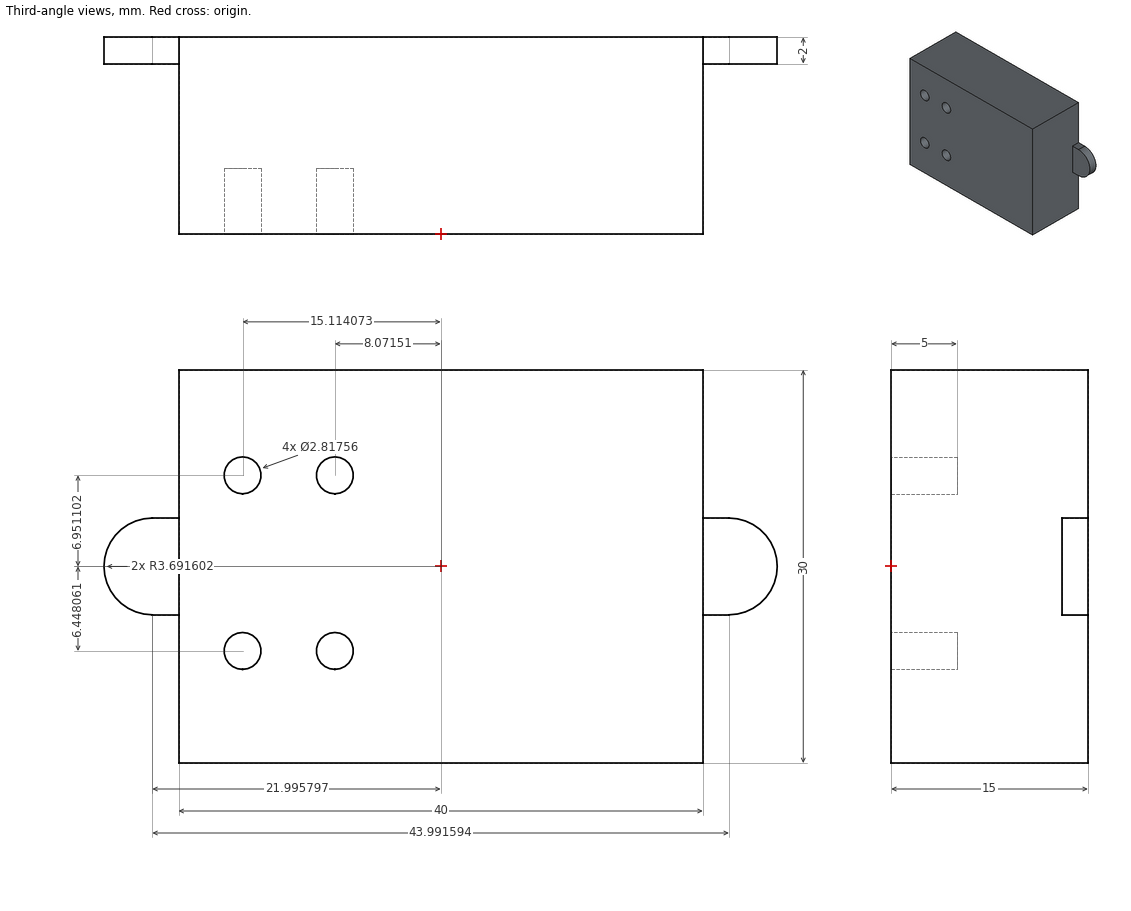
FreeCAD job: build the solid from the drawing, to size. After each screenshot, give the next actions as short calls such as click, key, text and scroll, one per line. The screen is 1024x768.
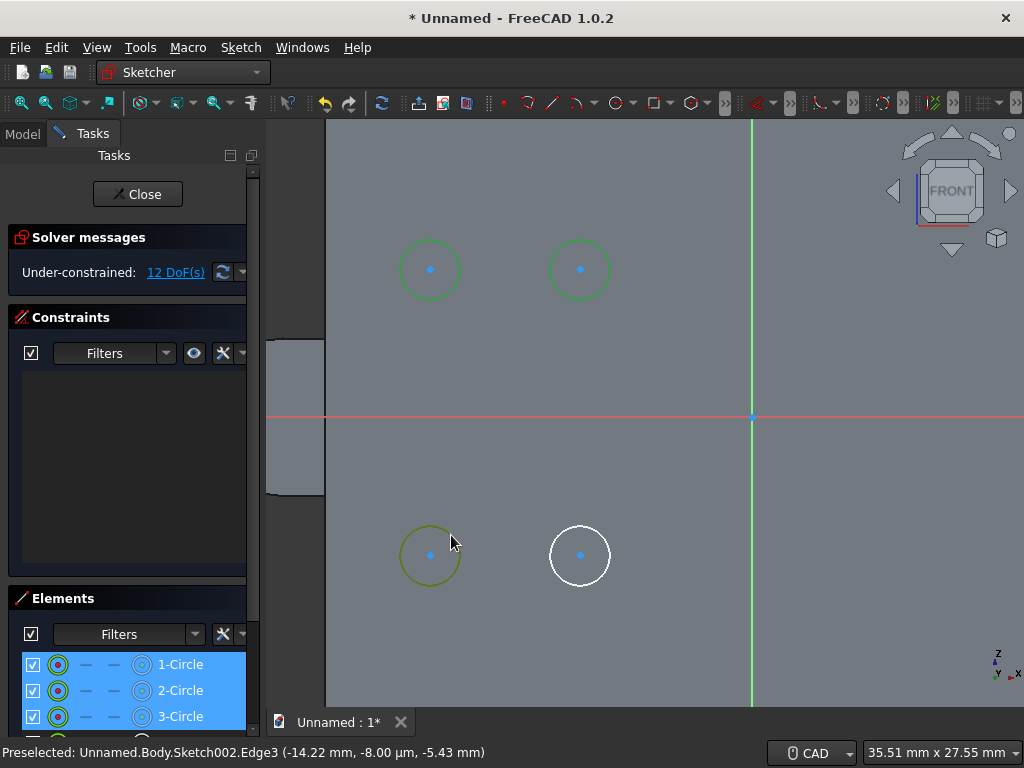
click(601, 535)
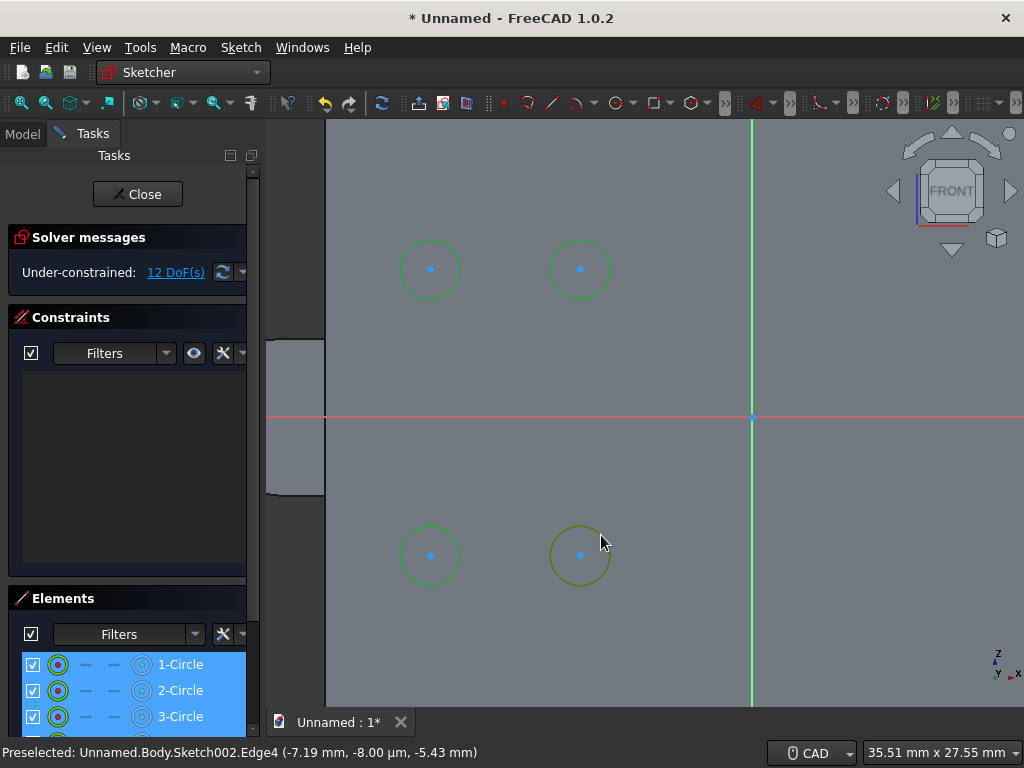
key(e)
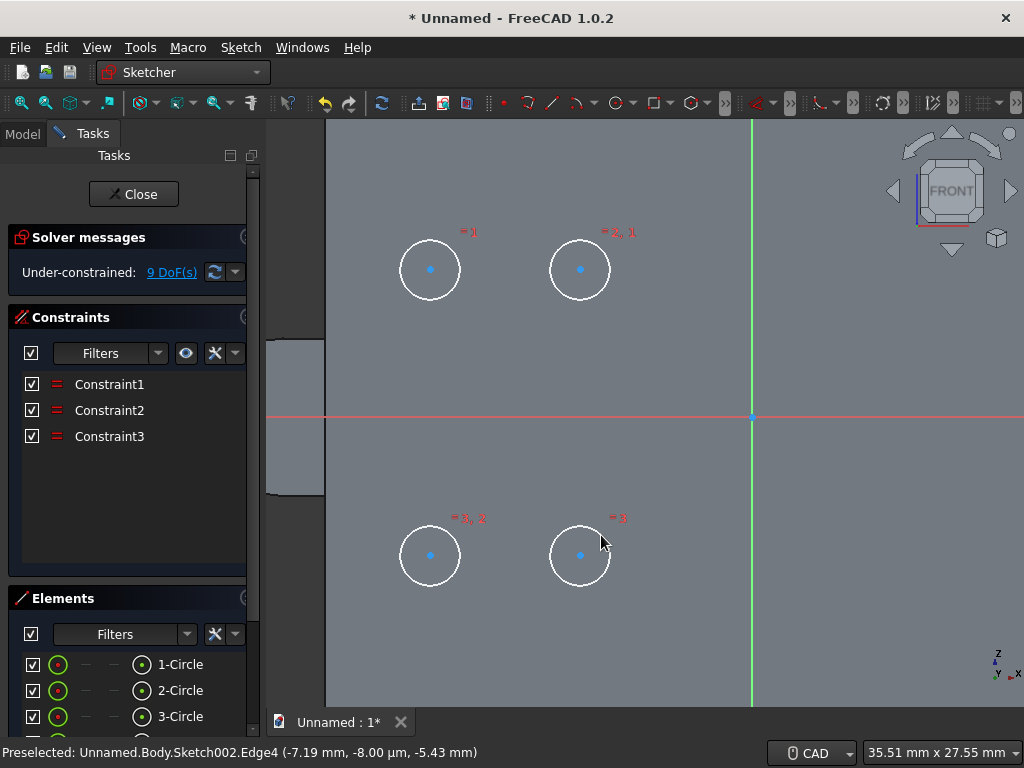
key(d)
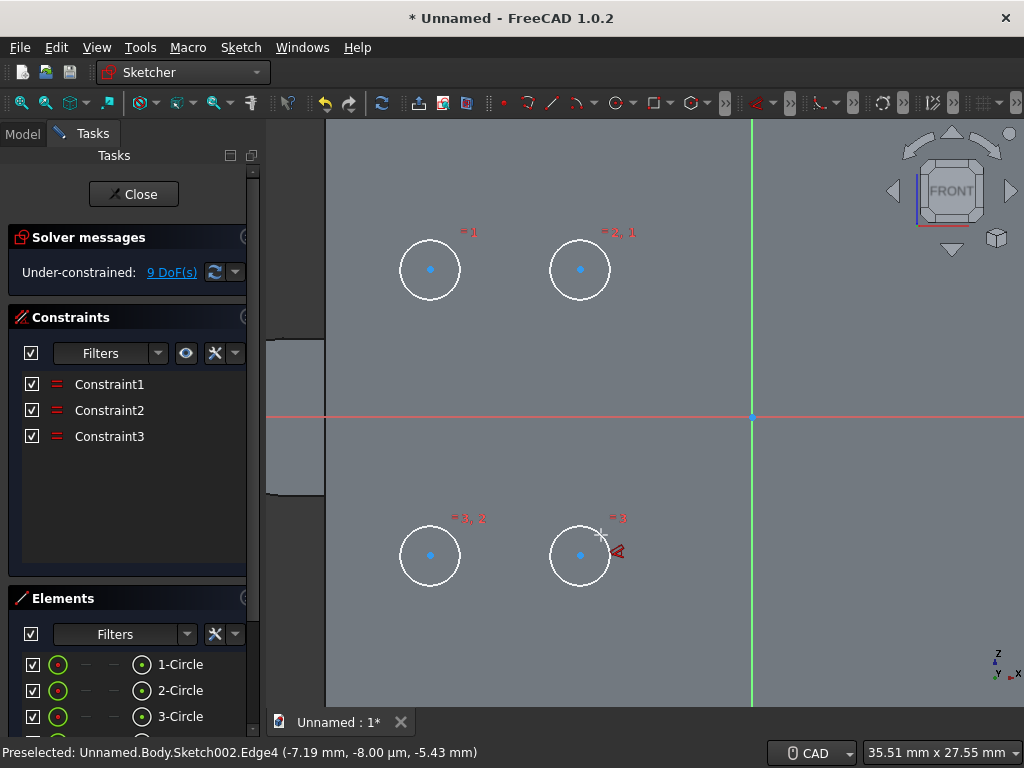
click(451, 249)
click(474, 226)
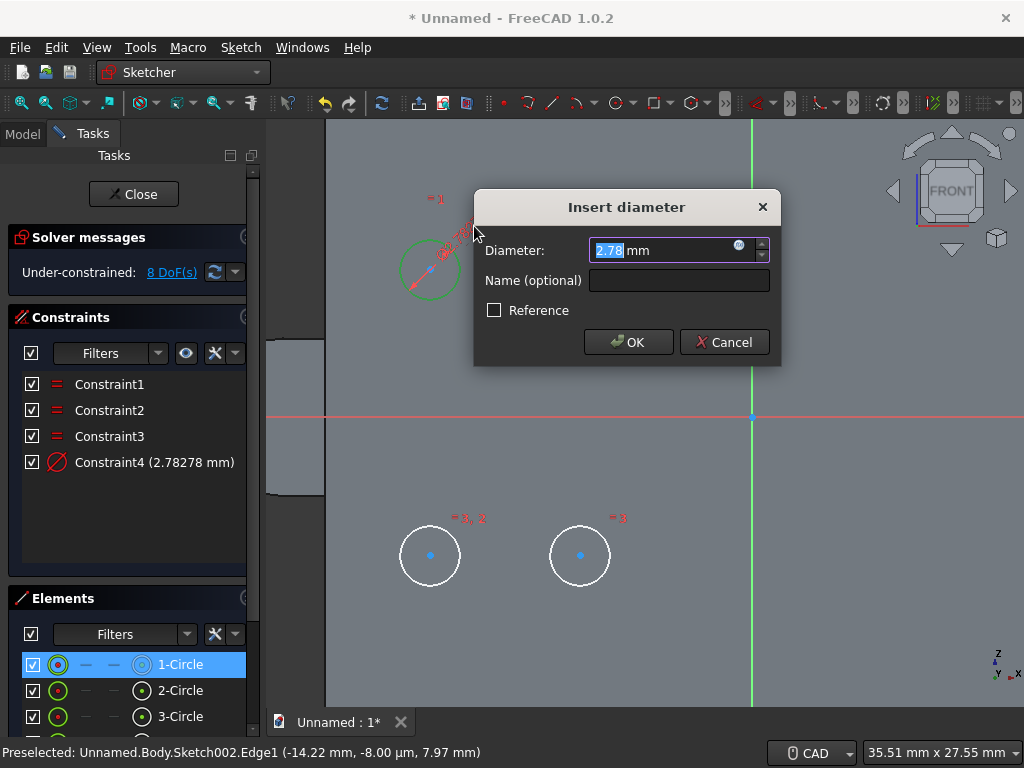
text(2.81756)
key(Return)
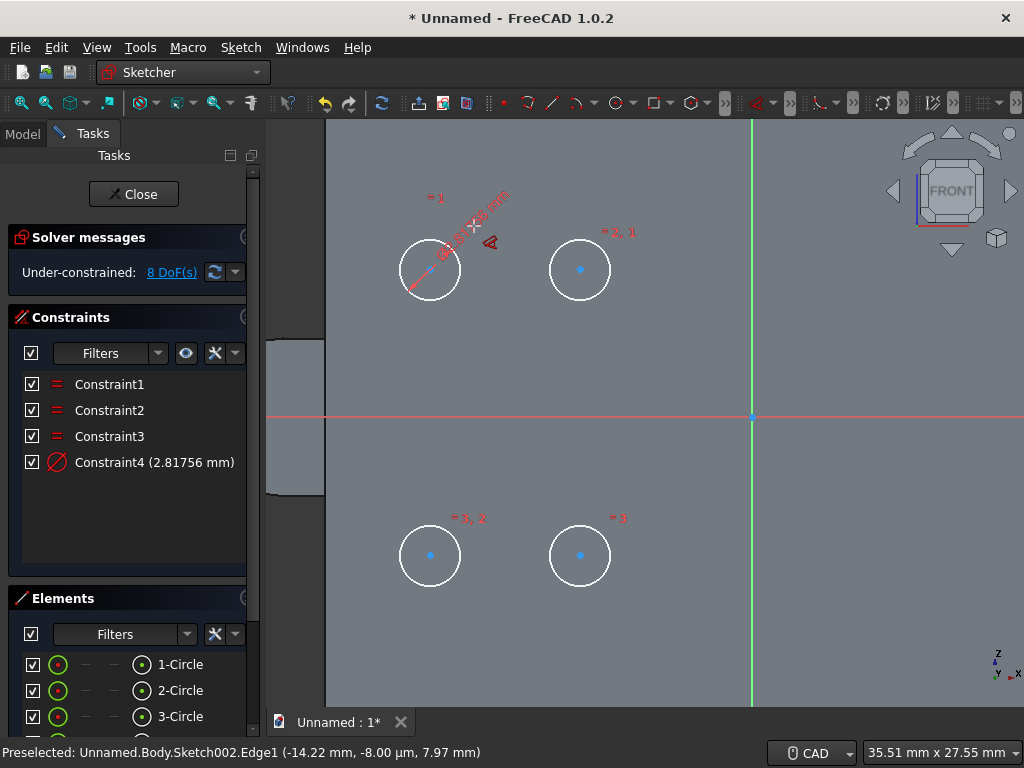
click(580, 270)
click(666, 236)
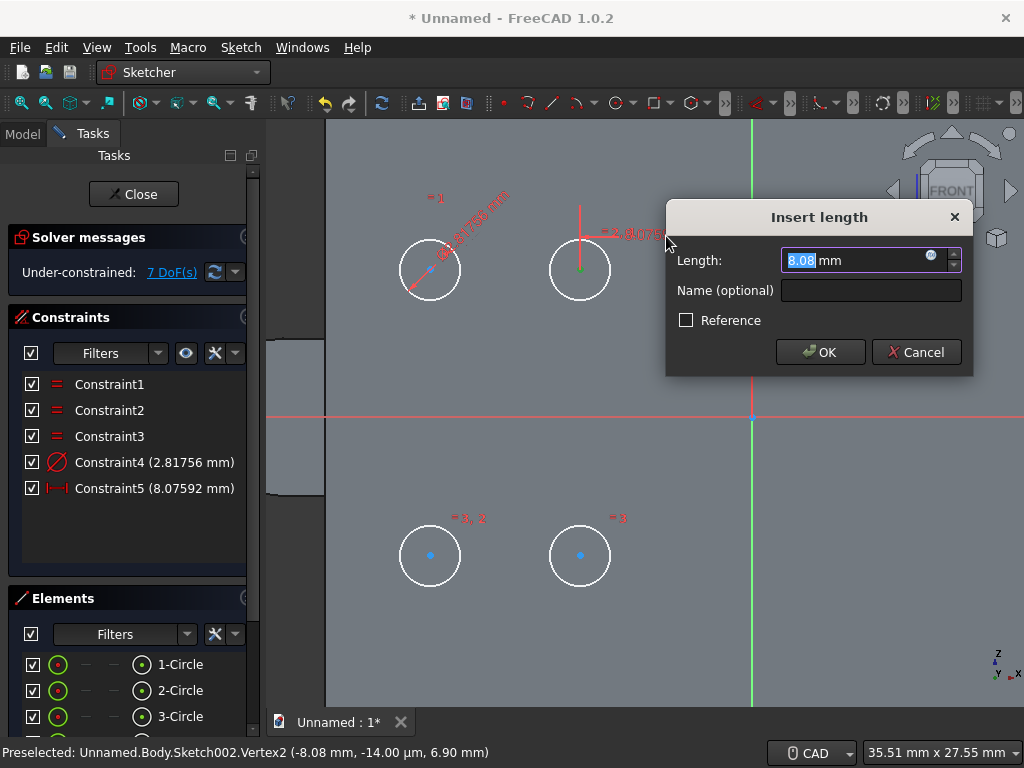
text(8.07151)
key(Return)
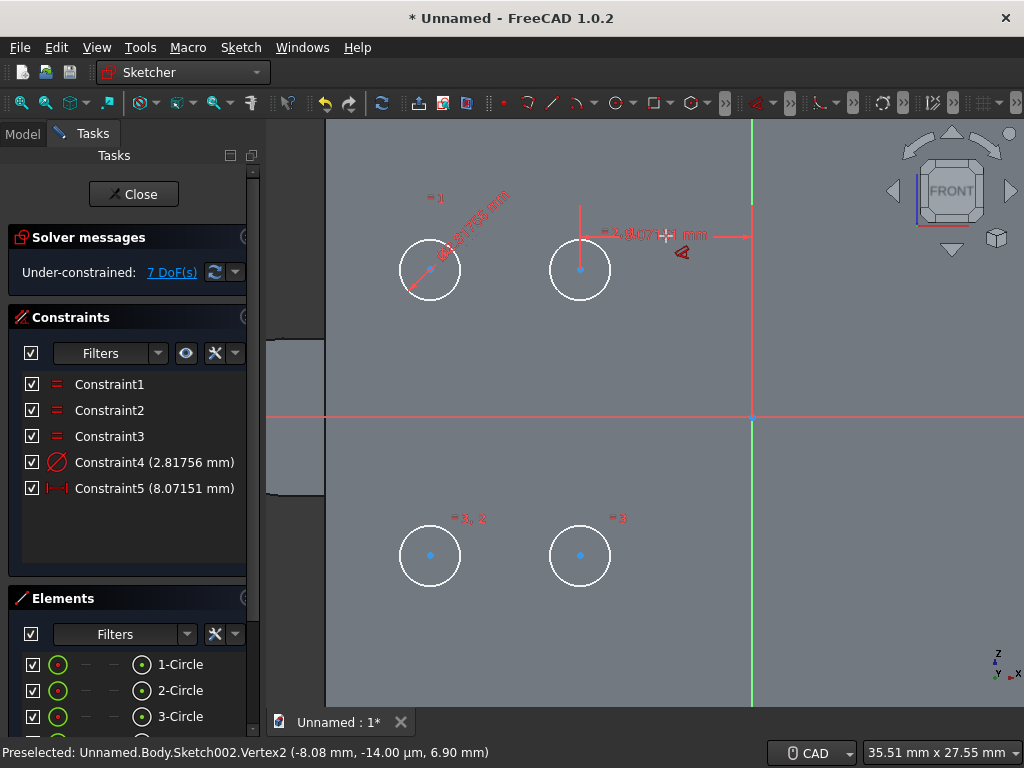
click(580, 556)
click(666, 590)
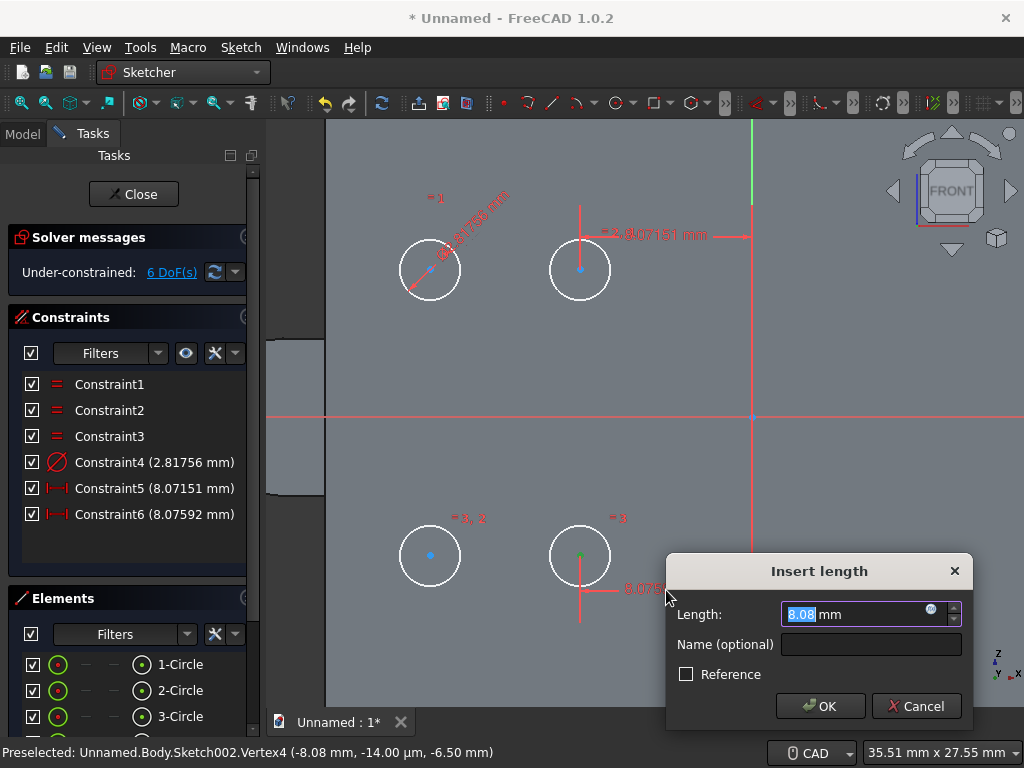
text(8.07151)
key(Return)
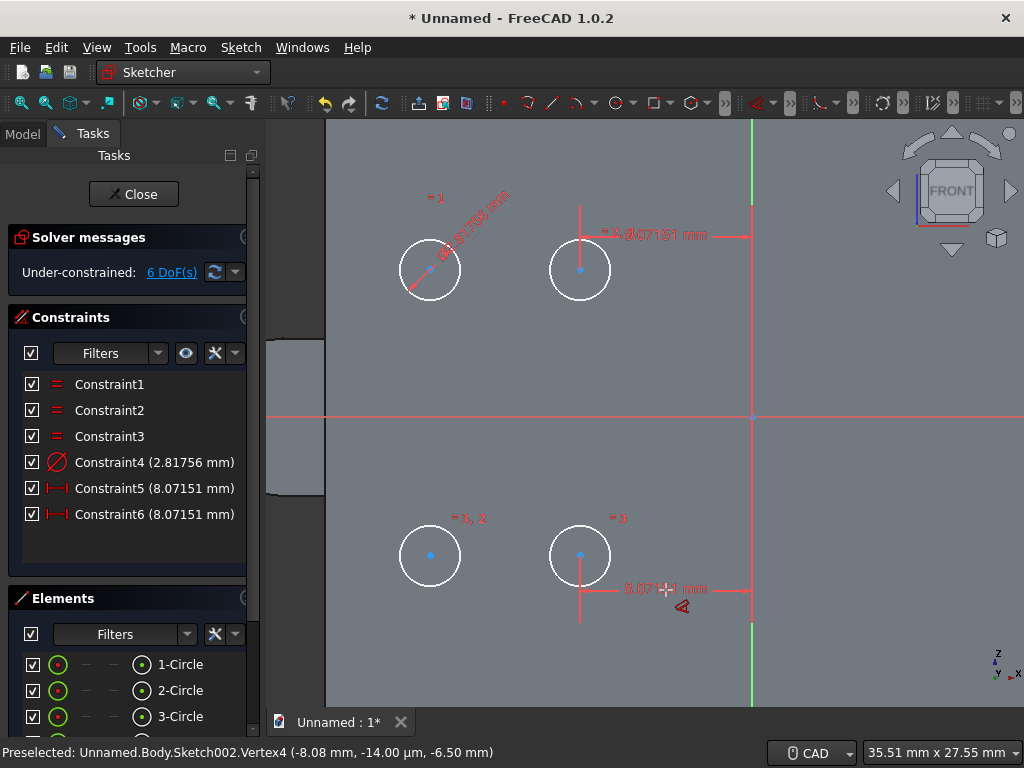
click(430, 270)
click(786, 344)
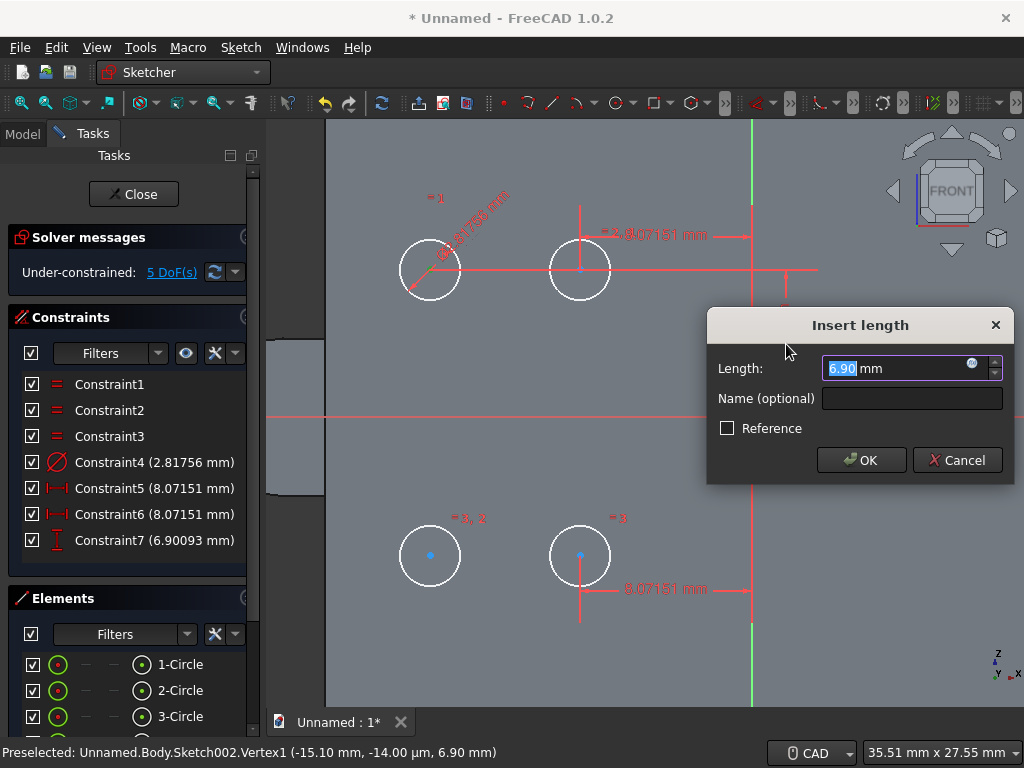
text(6.951102)
key(Return)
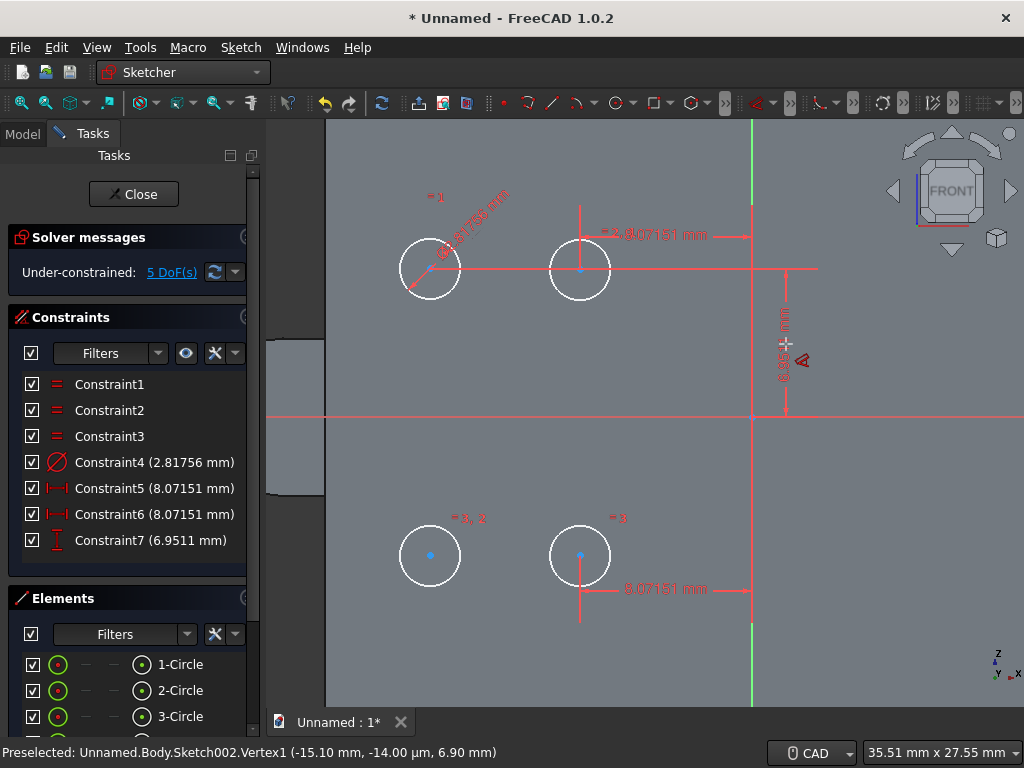
click(580, 270)
click(786, 310)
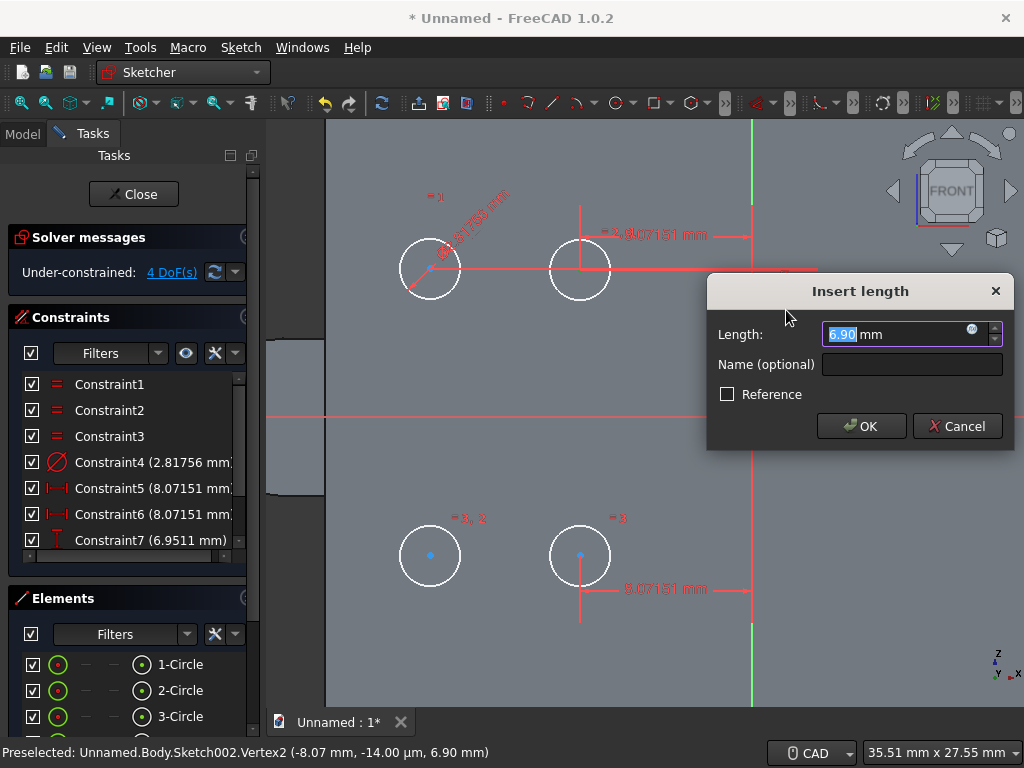
text(6.951102)
key(Return)